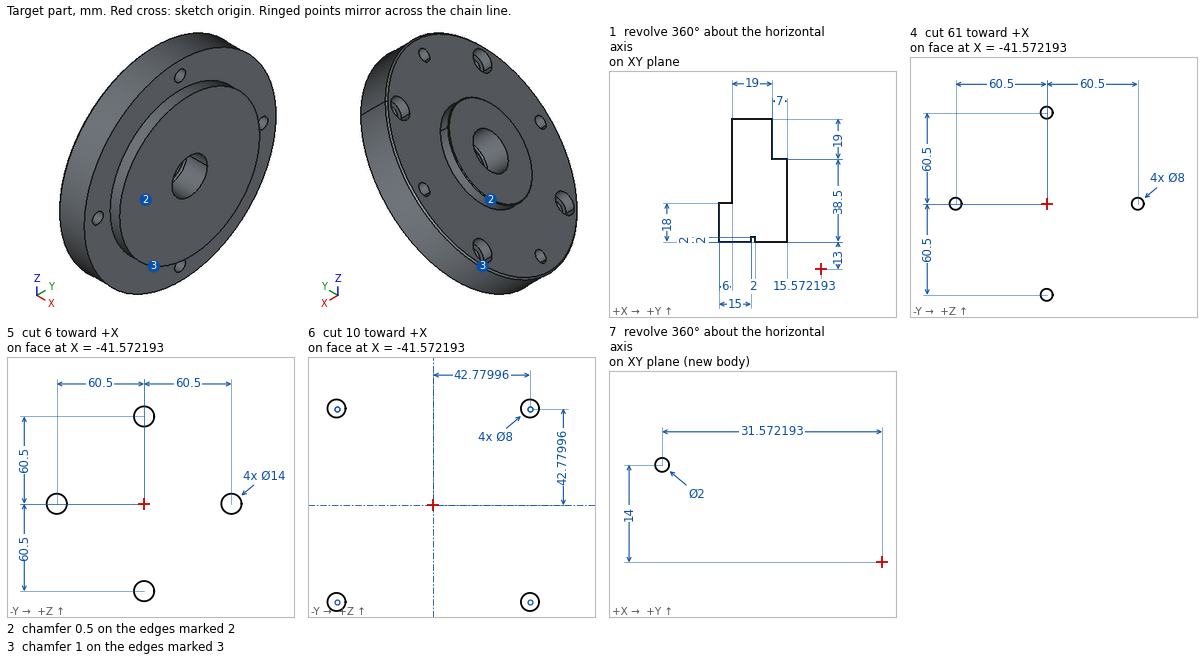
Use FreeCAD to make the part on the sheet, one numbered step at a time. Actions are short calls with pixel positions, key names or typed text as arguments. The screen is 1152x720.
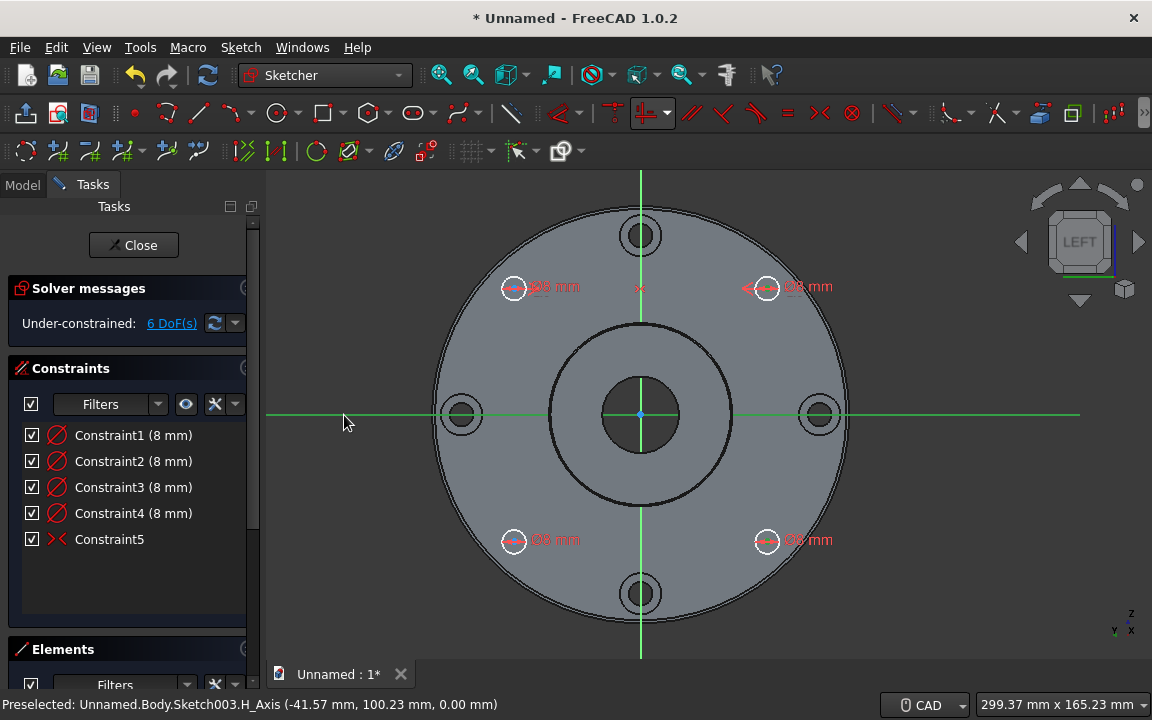
click(820, 114)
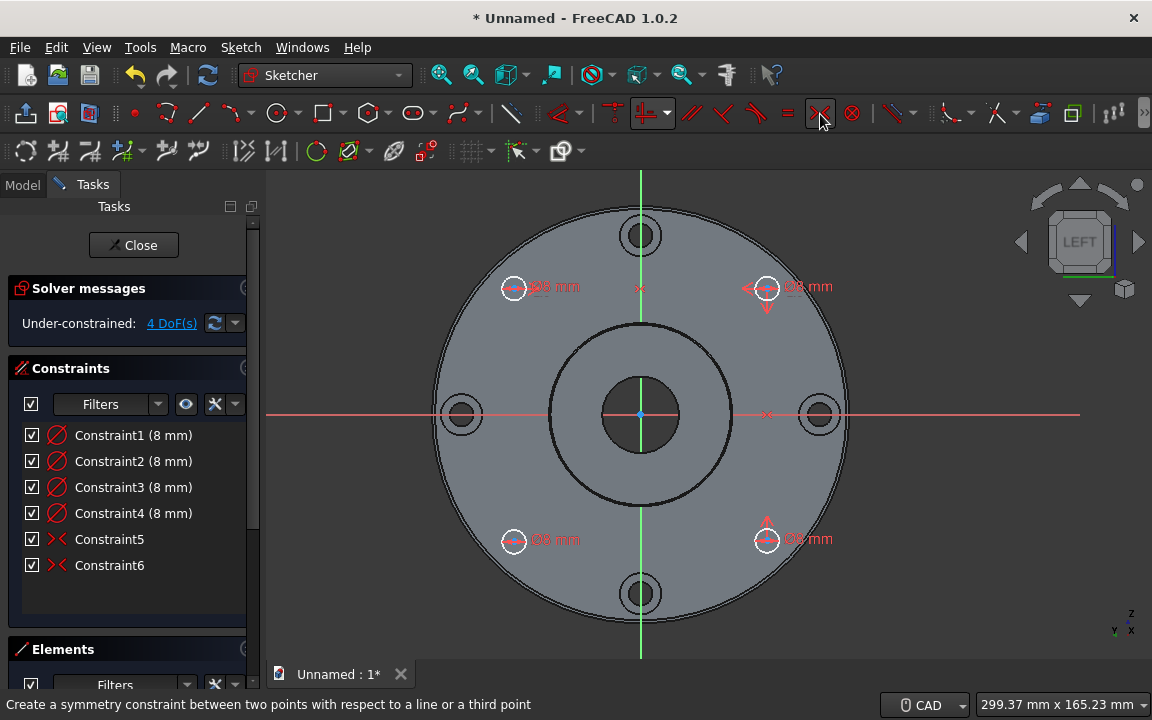
click(514, 289)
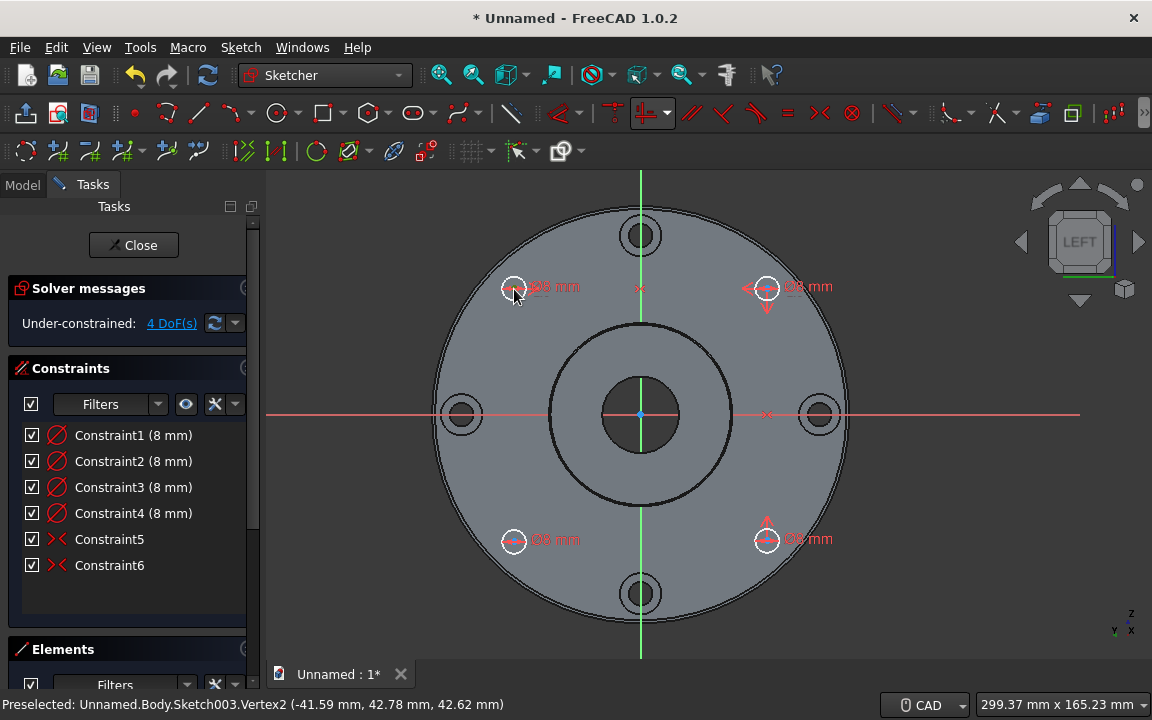
click(514, 542)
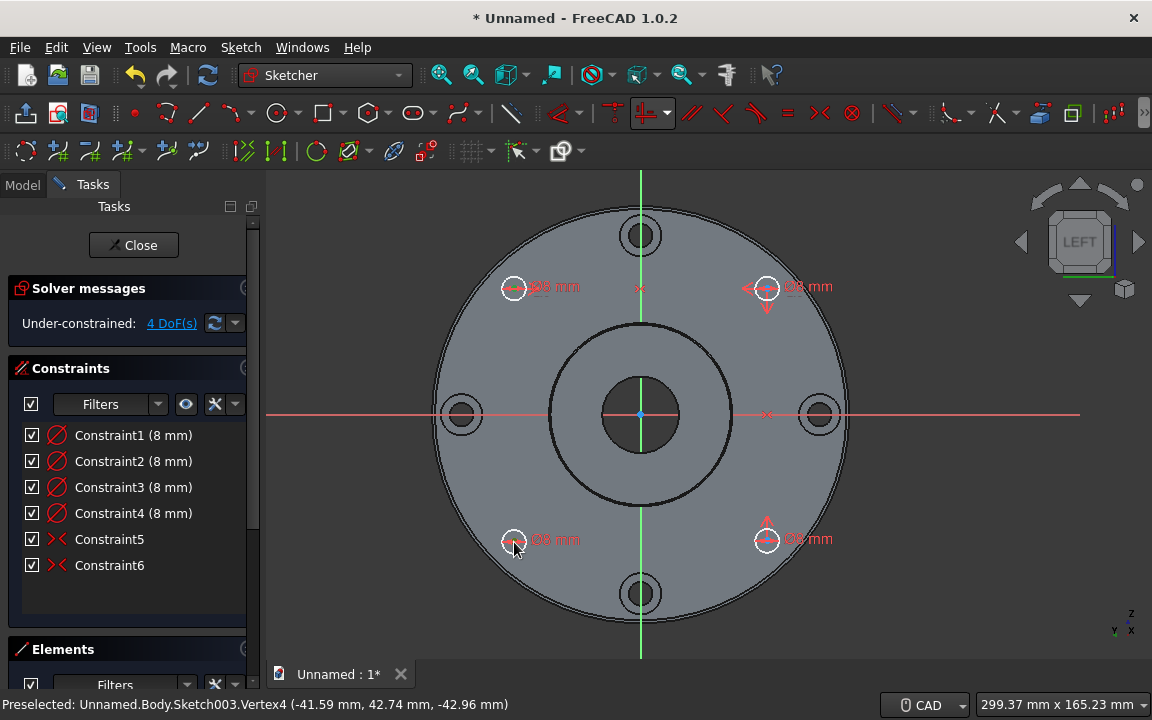
click(344, 415)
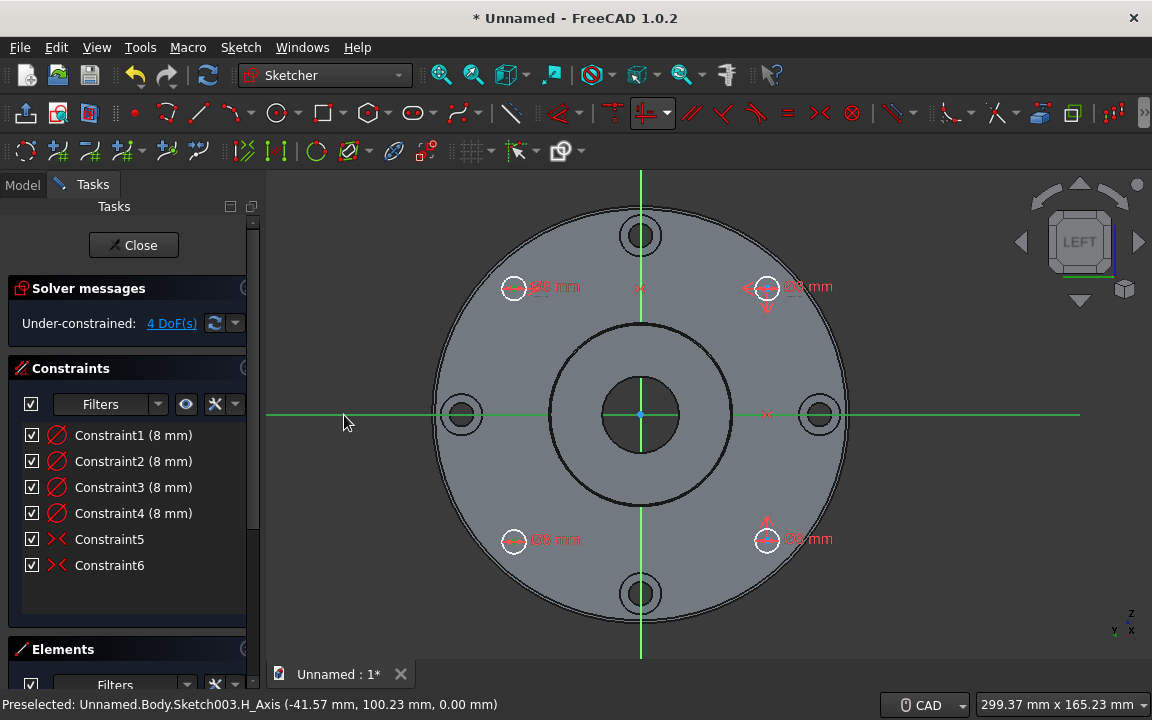
click(820, 114)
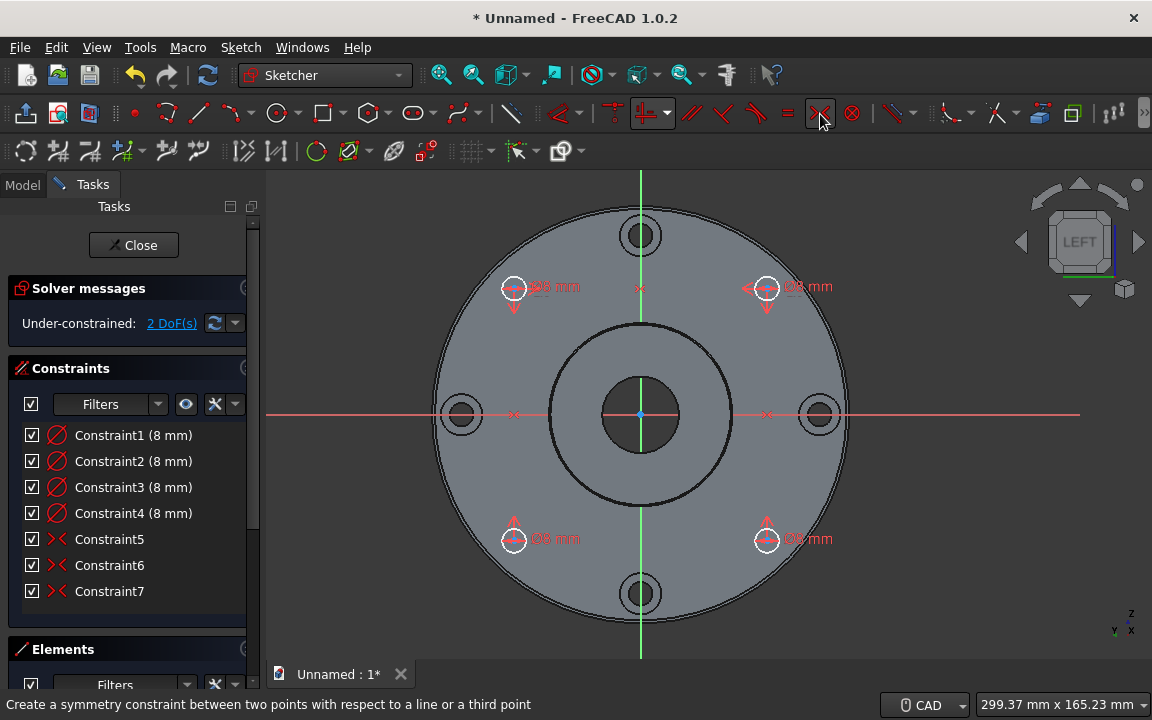
click(558, 114)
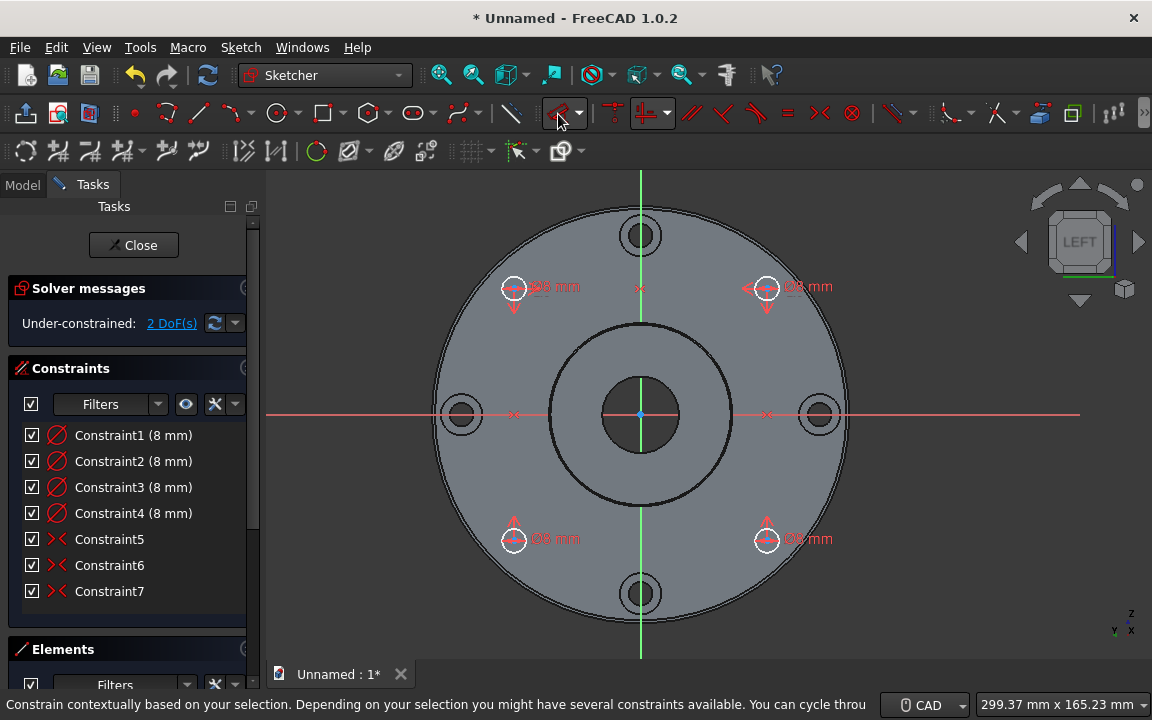
click(767, 289)
click(704, 255)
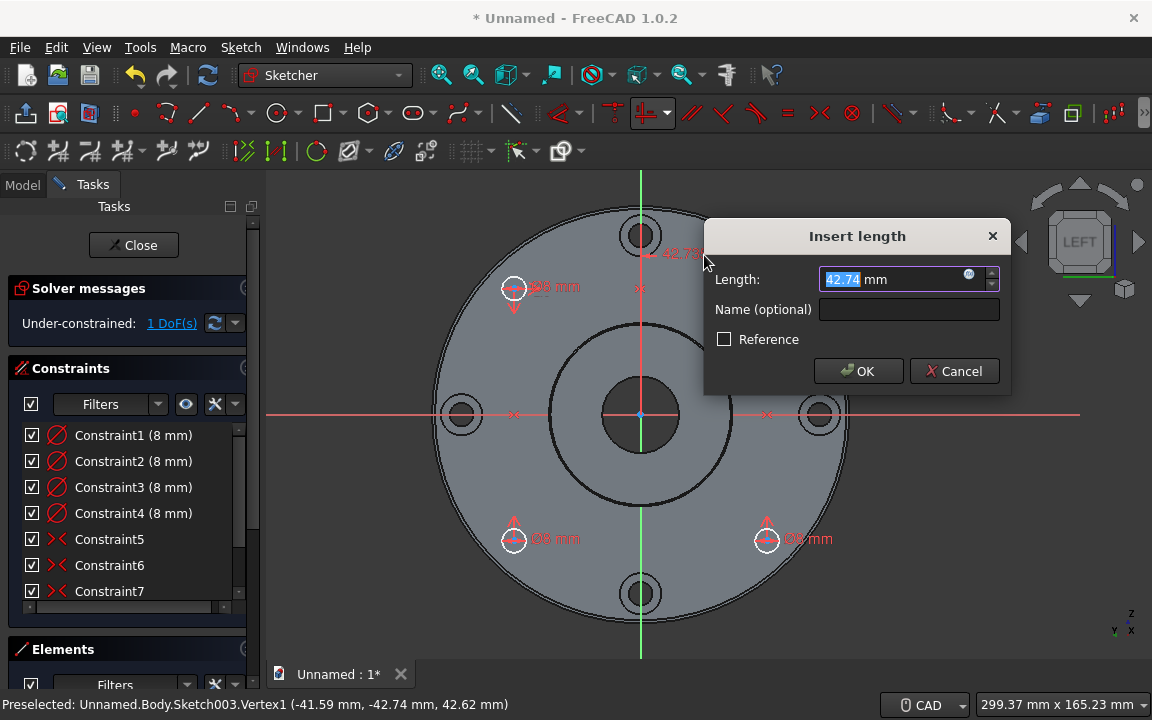
text(42.77996)
key(Return)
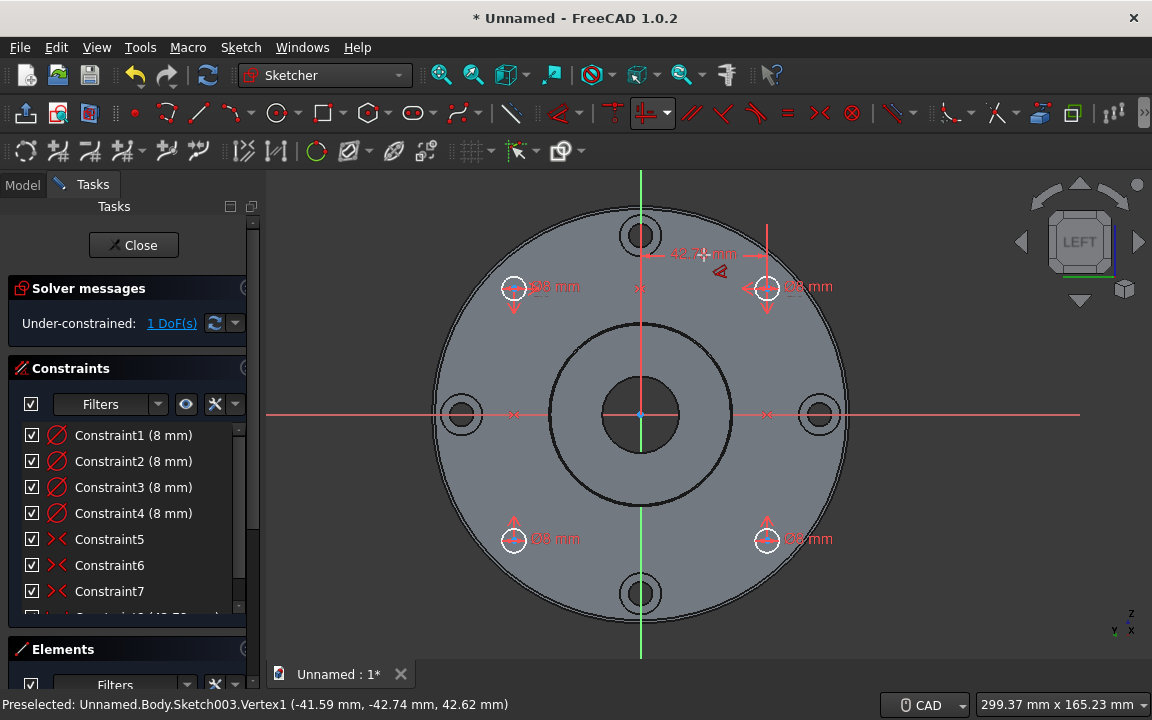
click(767, 289)
click(801, 352)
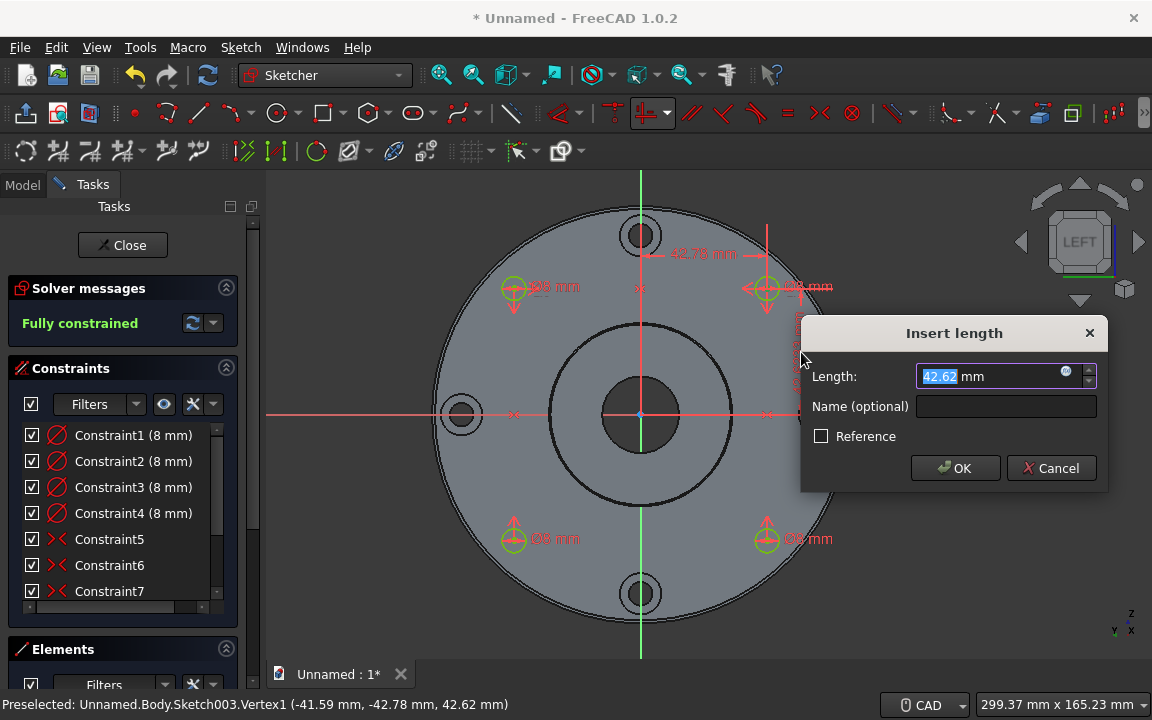
text(42.77996)
key(Return)
key(Escape)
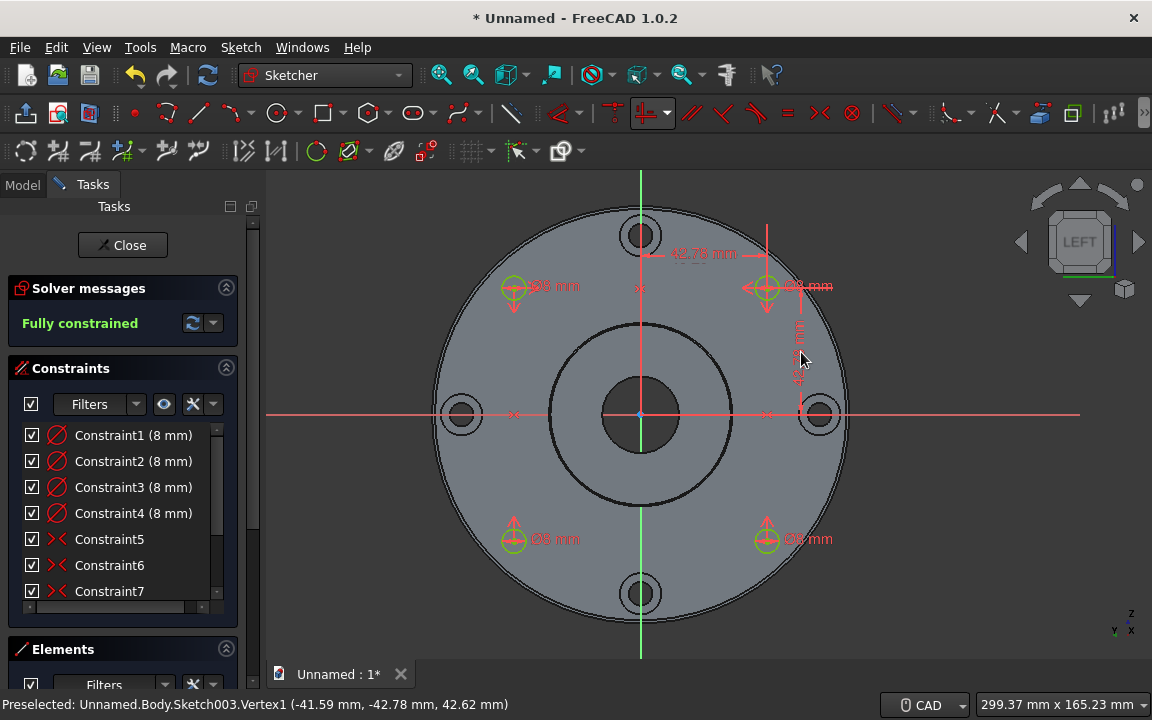
click(123, 245)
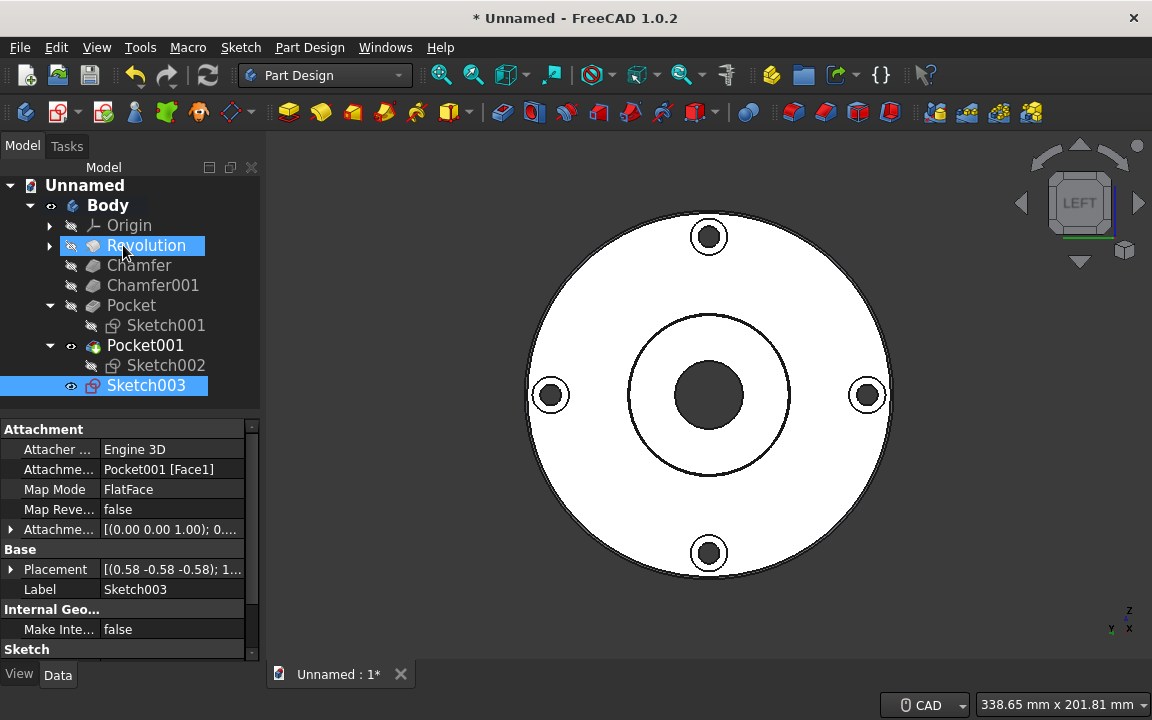
click(504, 112)